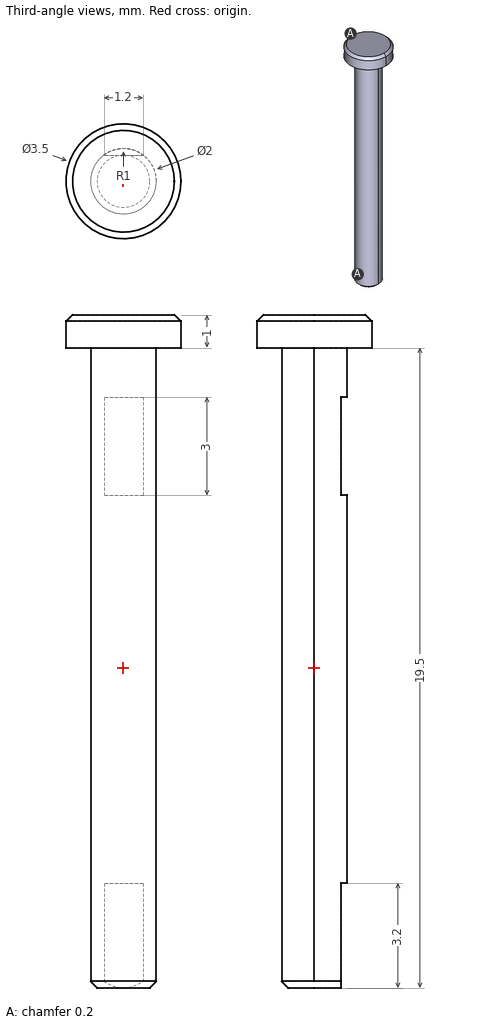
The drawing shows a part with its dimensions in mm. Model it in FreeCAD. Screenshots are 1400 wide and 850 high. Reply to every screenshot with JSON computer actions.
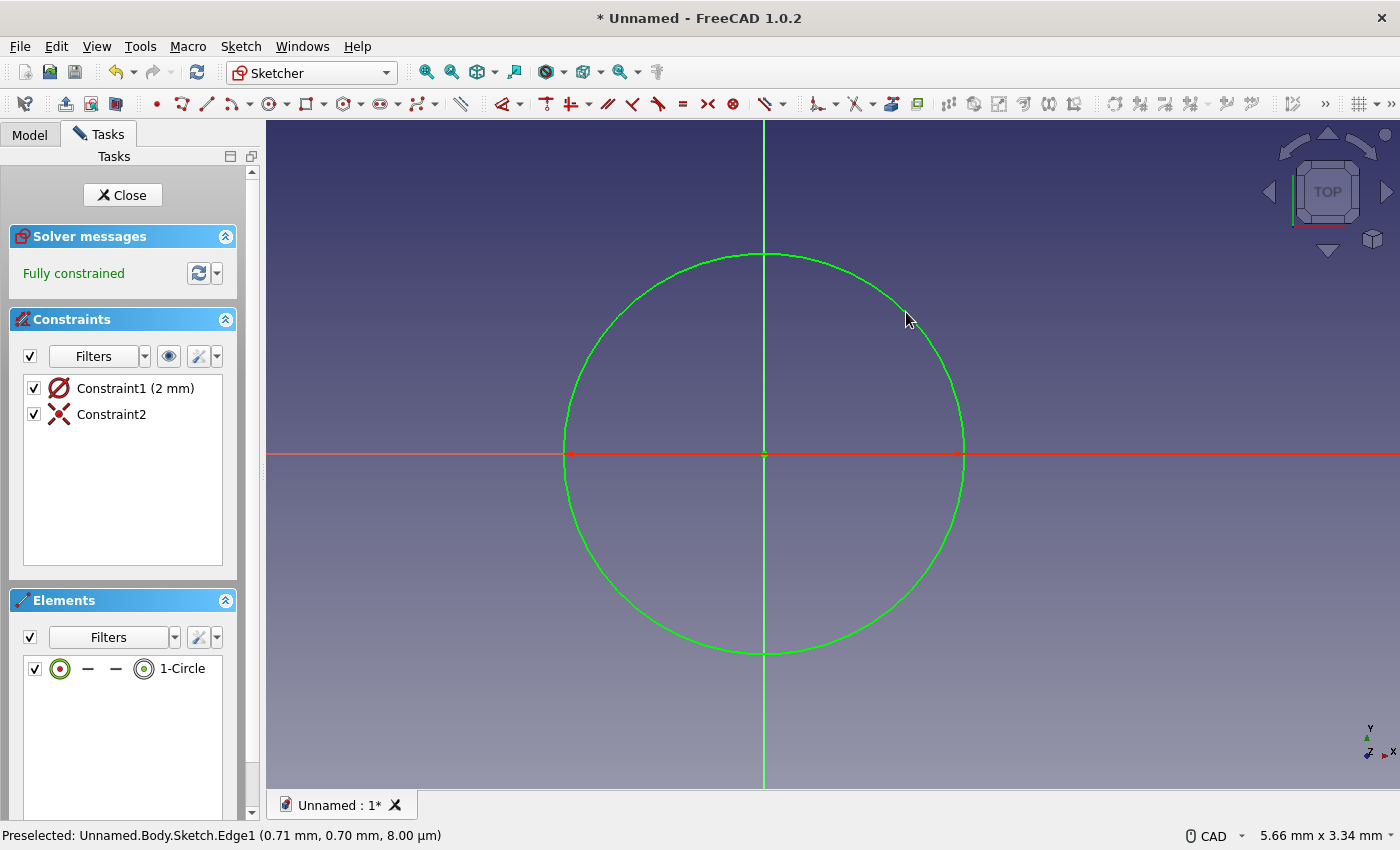
{"action": "left_click", "coordinate": [123, 195]}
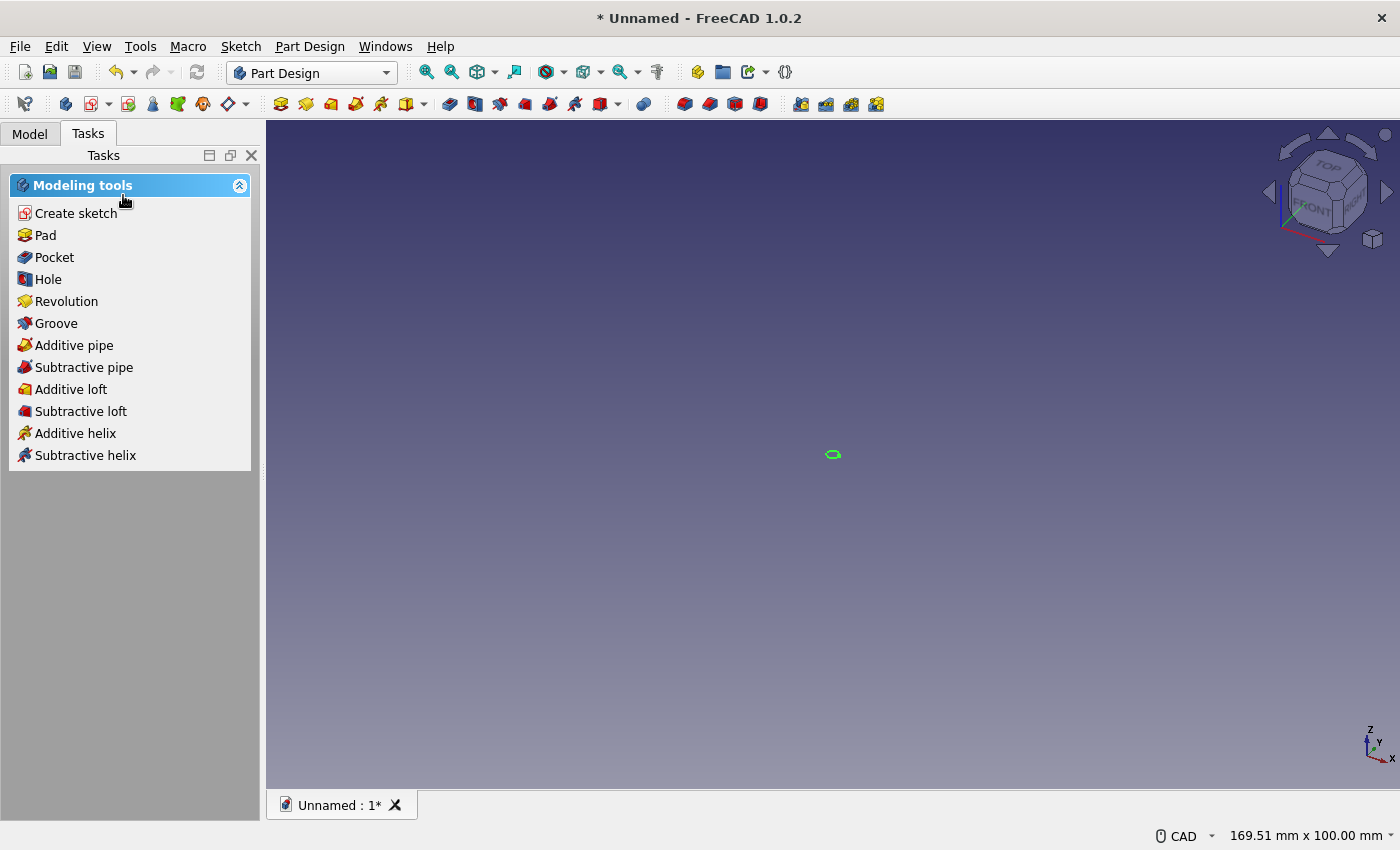
{"action": "left_click", "coordinate": [281, 104]}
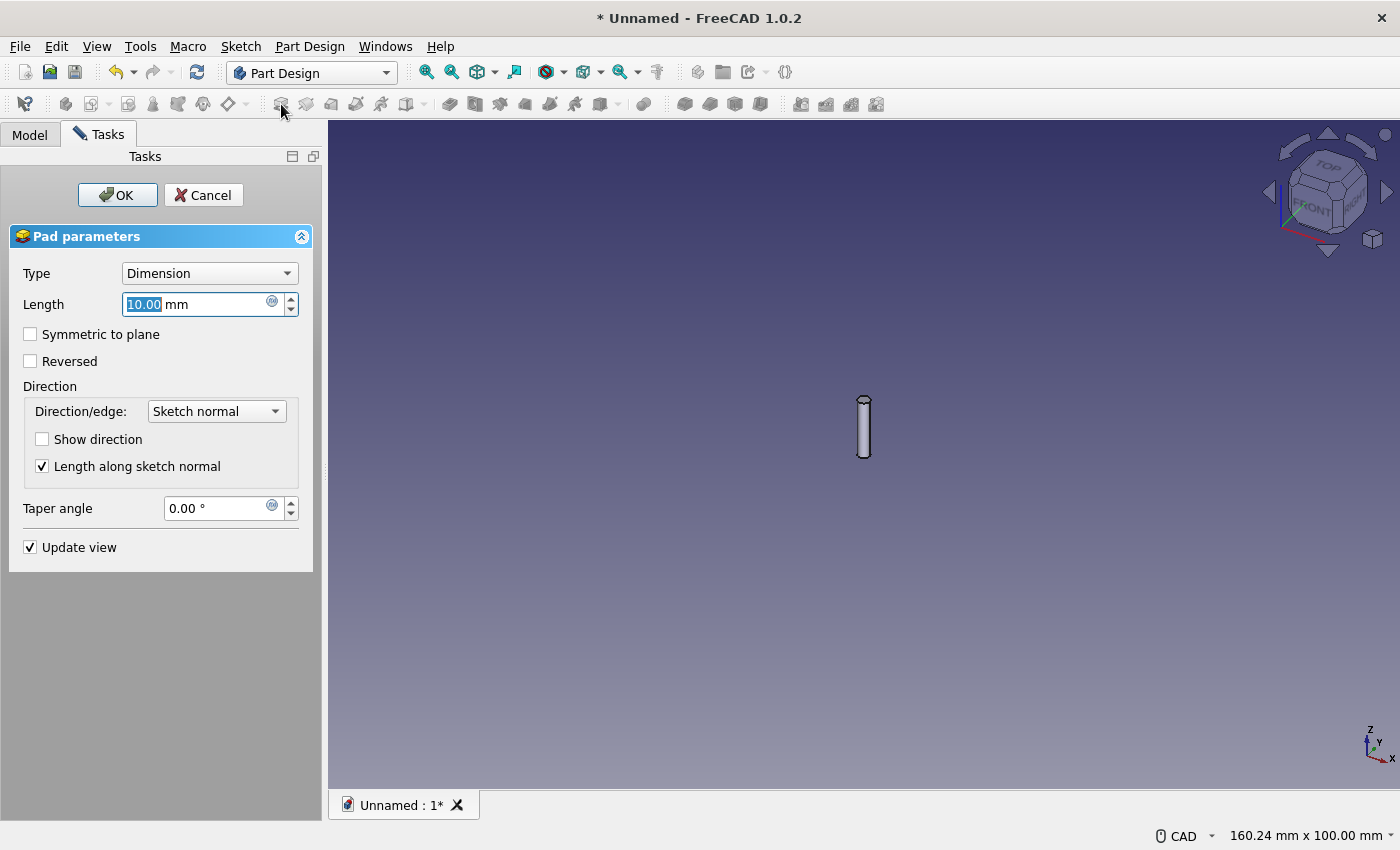
{"action": "type", "text": "19.5"}
{"action": "key", "text": "Tab"}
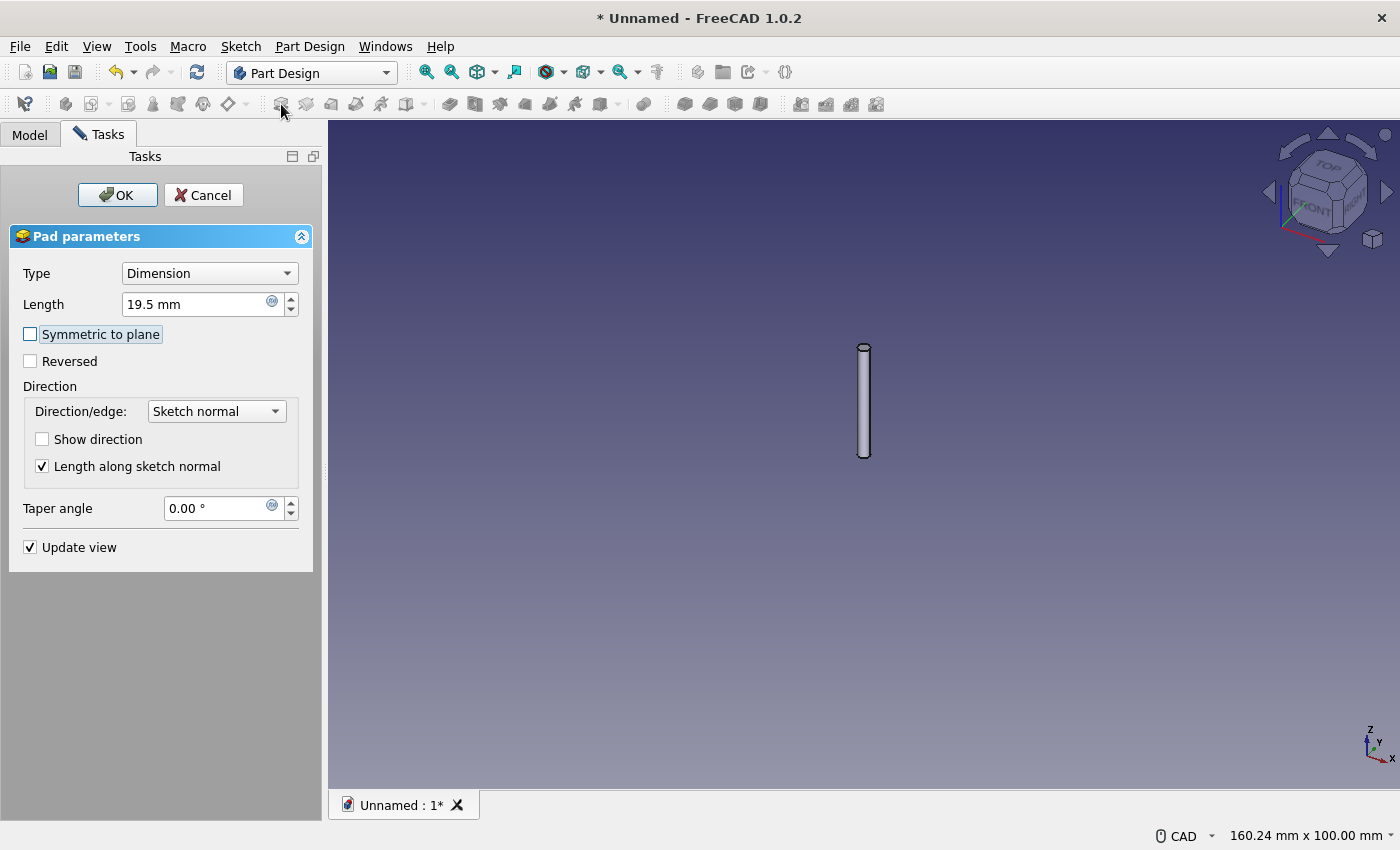
{"action": "left_click", "coordinate": [31, 334]}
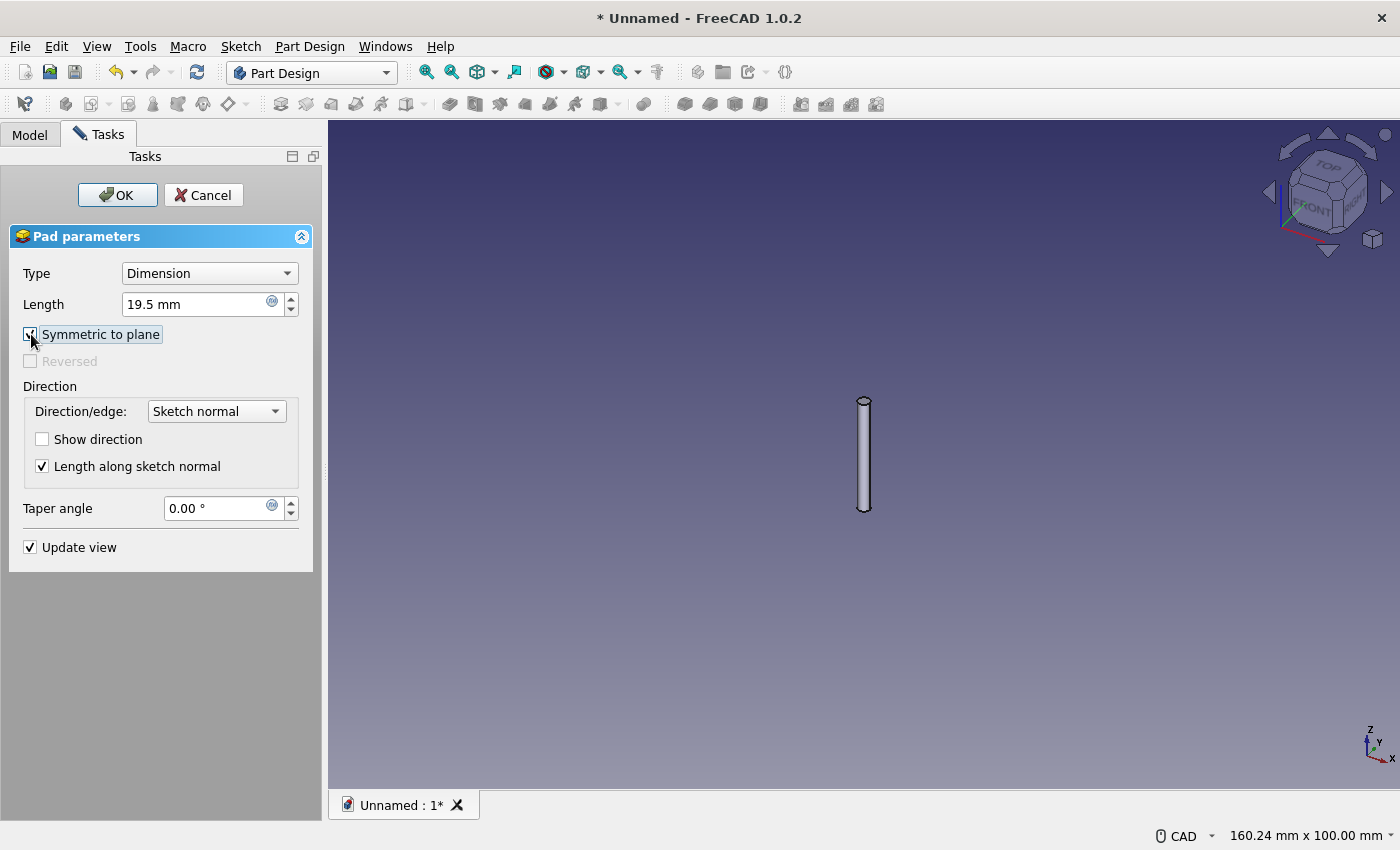
{"action": "left_click", "coordinate": [118, 195]}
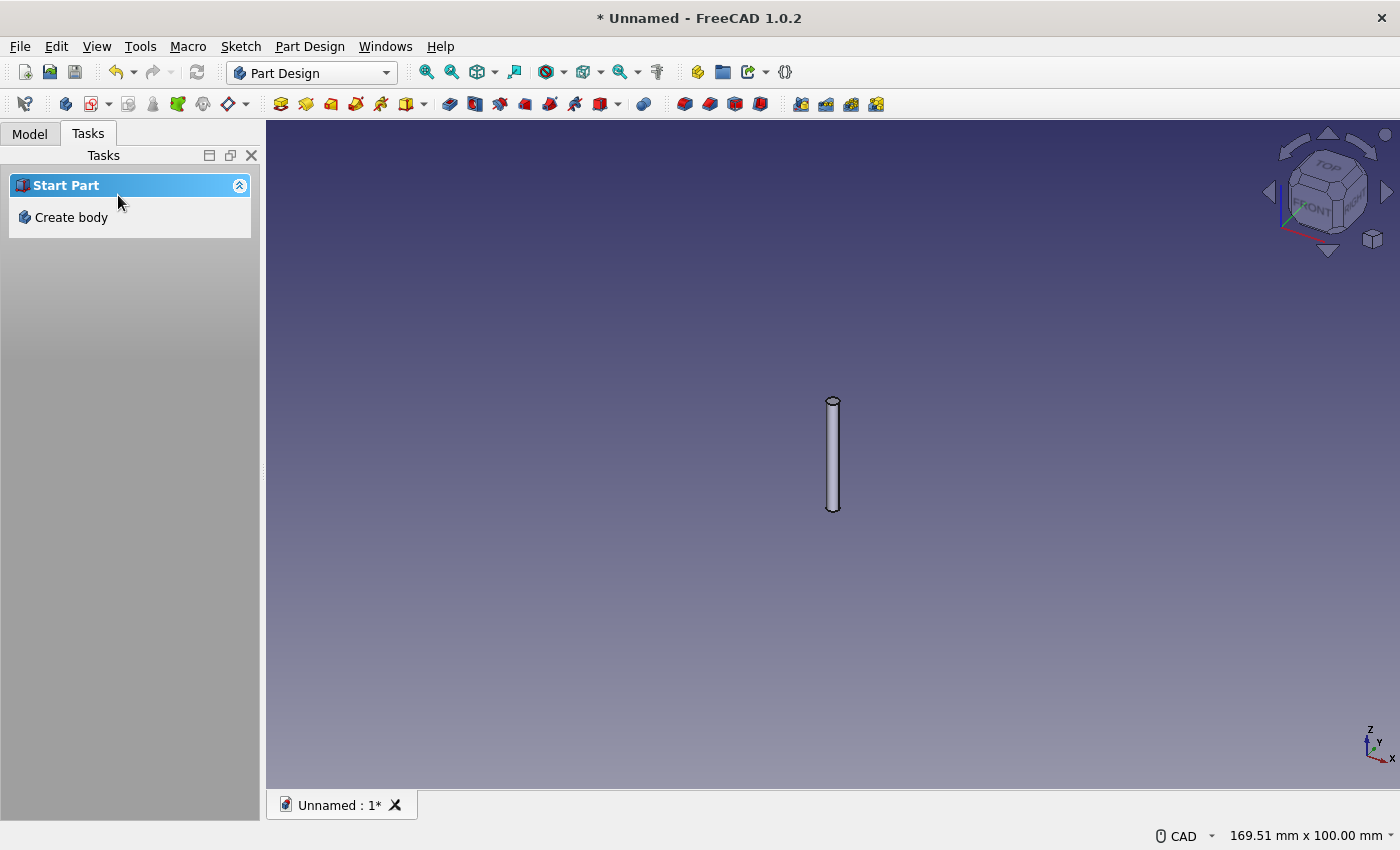
{"action": "left_click", "coordinate": [427, 72]}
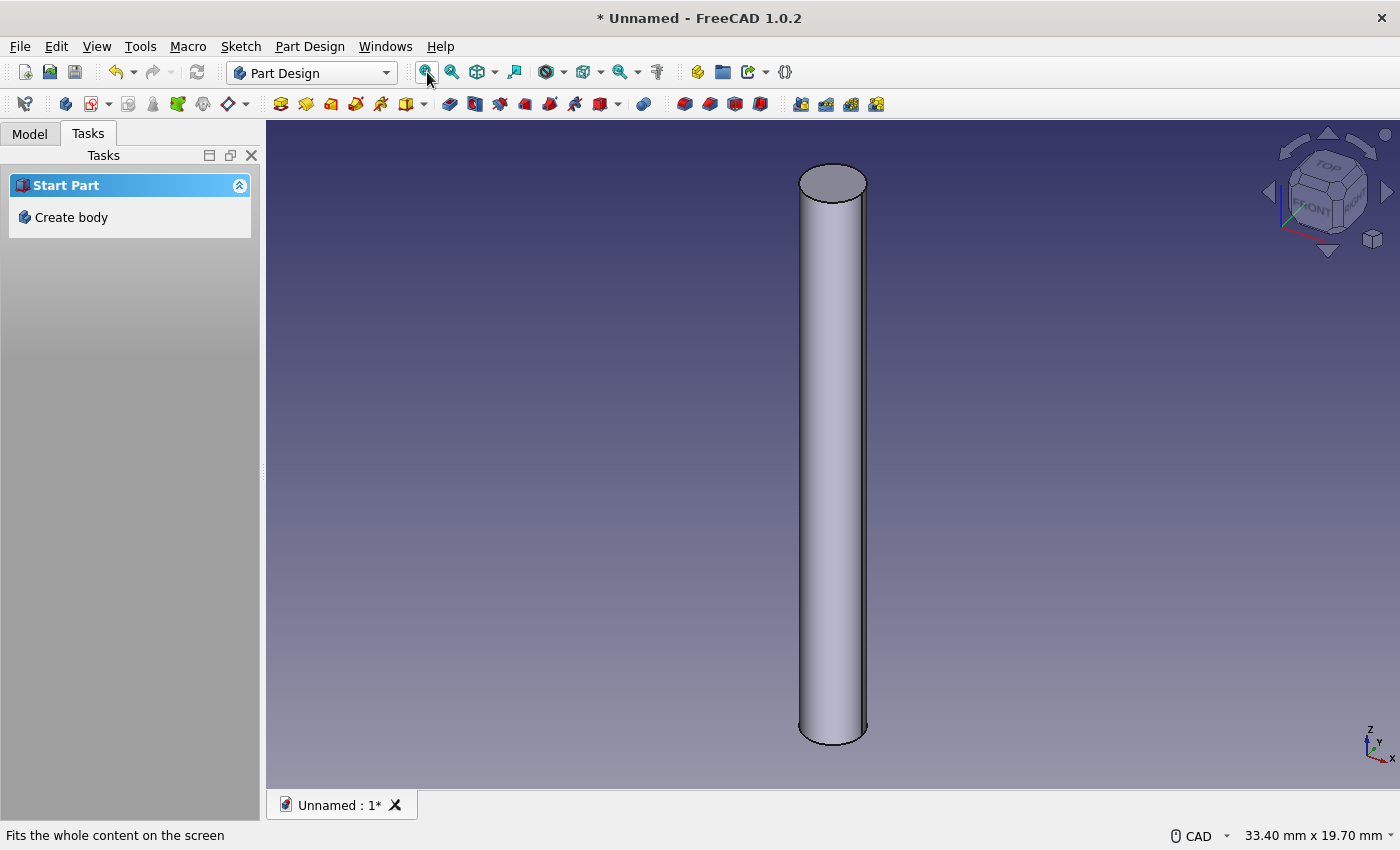
{"action": "left_click", "coordinate": [833, 182]}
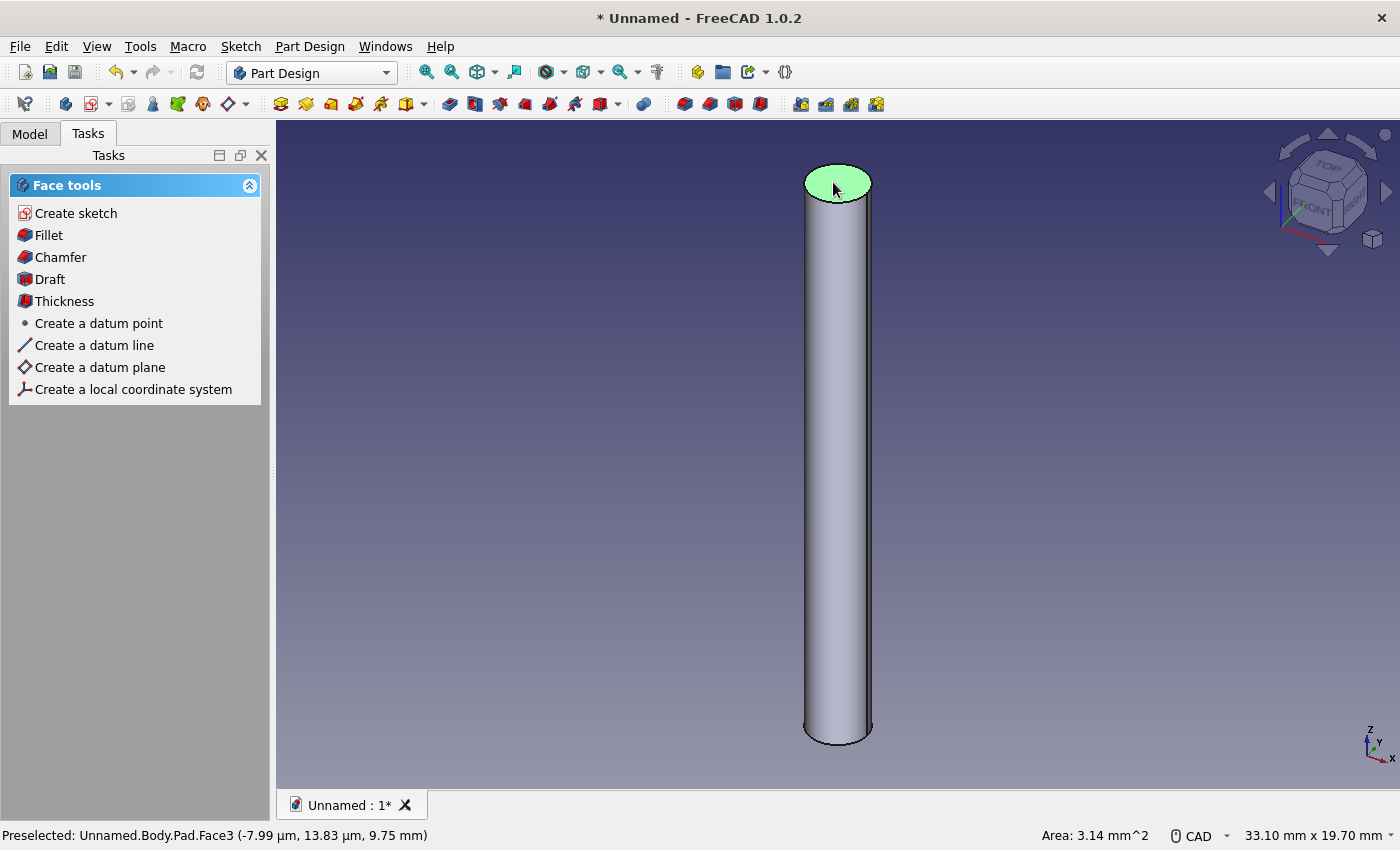
{"action": "left_click", "coordinate": [90, 104]}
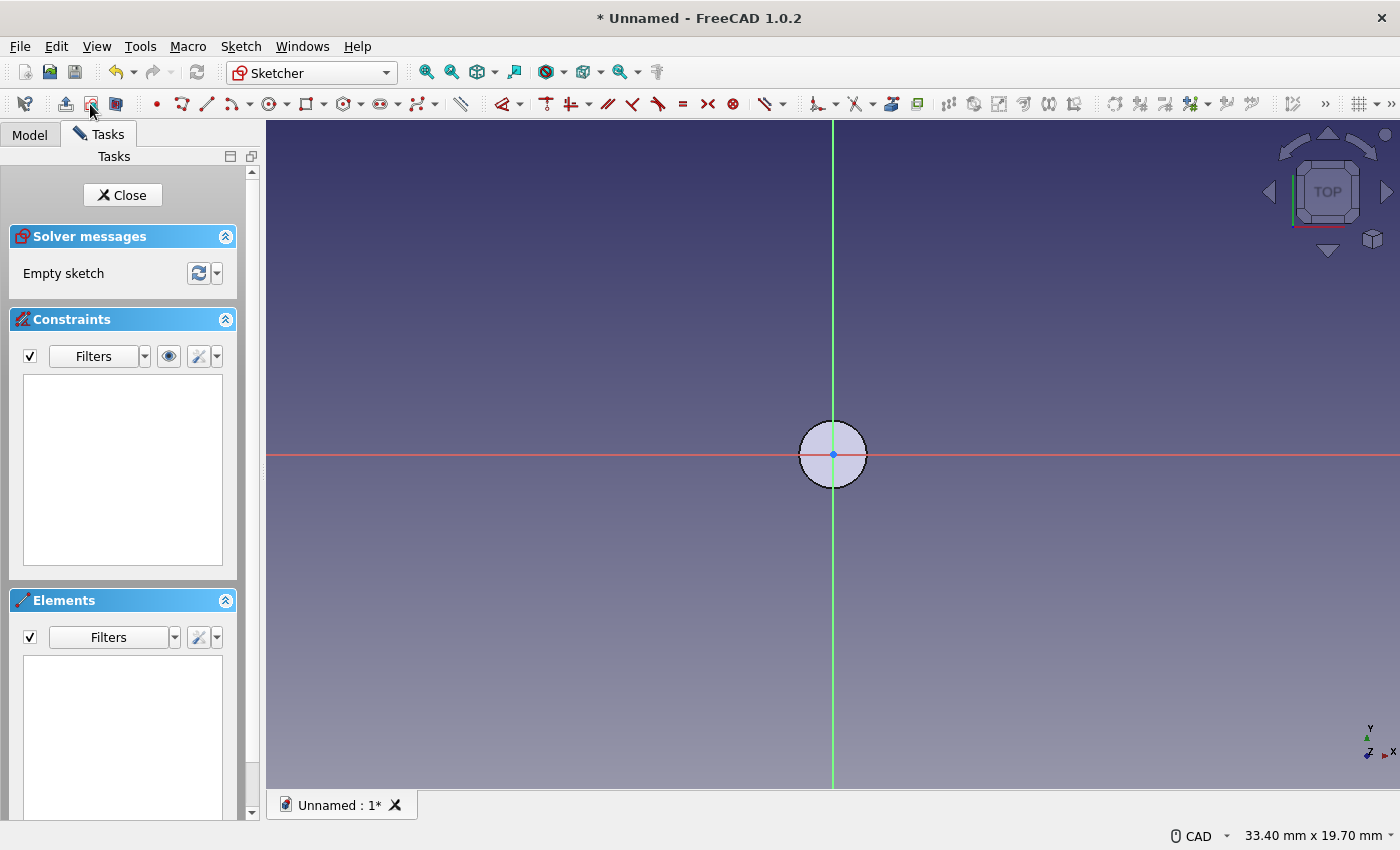
{"action": "scroll", "coordinate": [863, 455], "scroll_direction": "up", "scroll_amount": 6}